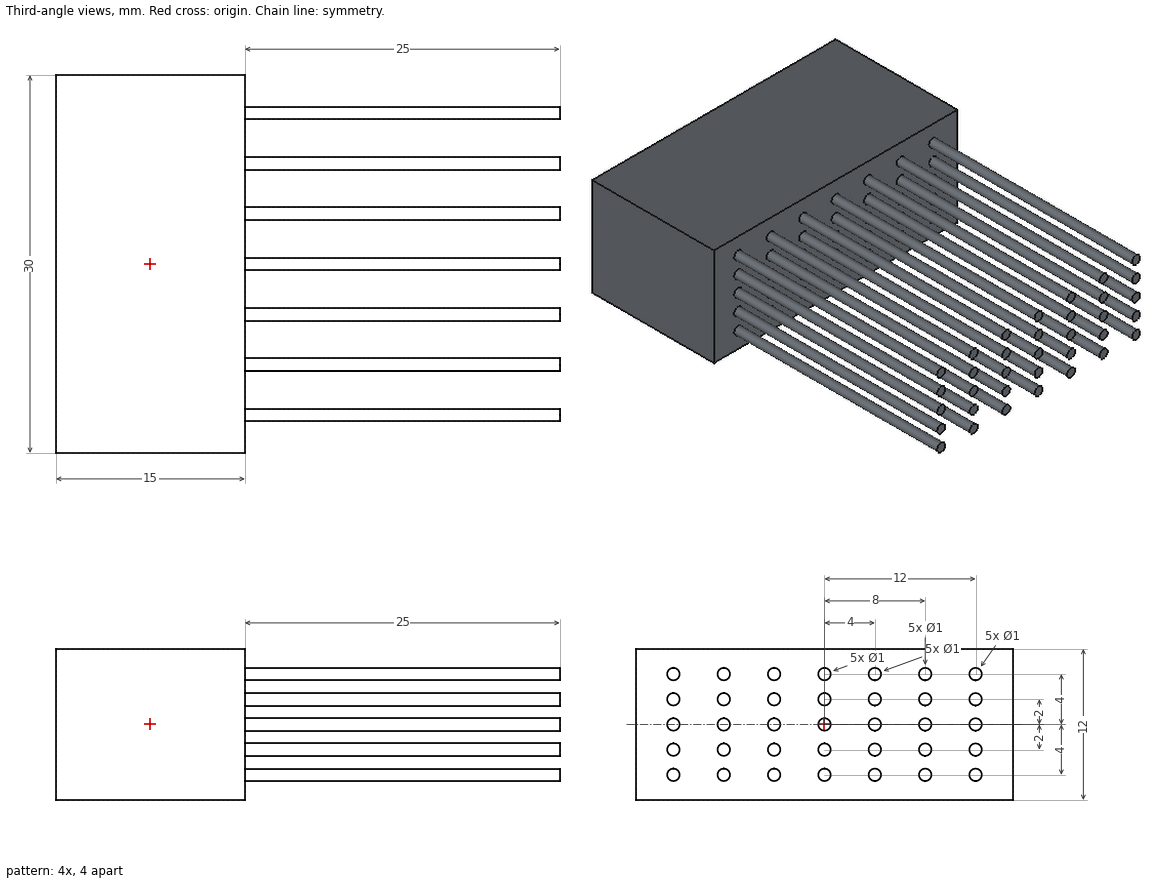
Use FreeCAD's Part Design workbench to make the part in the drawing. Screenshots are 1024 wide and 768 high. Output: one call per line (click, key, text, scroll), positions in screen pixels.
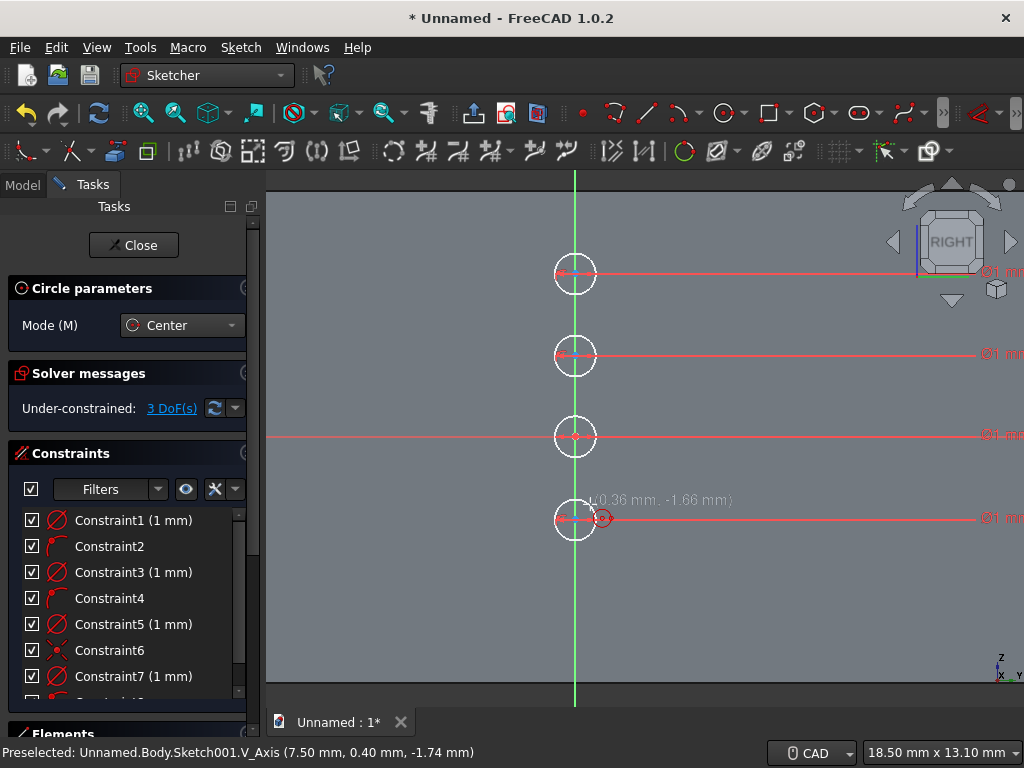
click(575, 601)
move(590, 586)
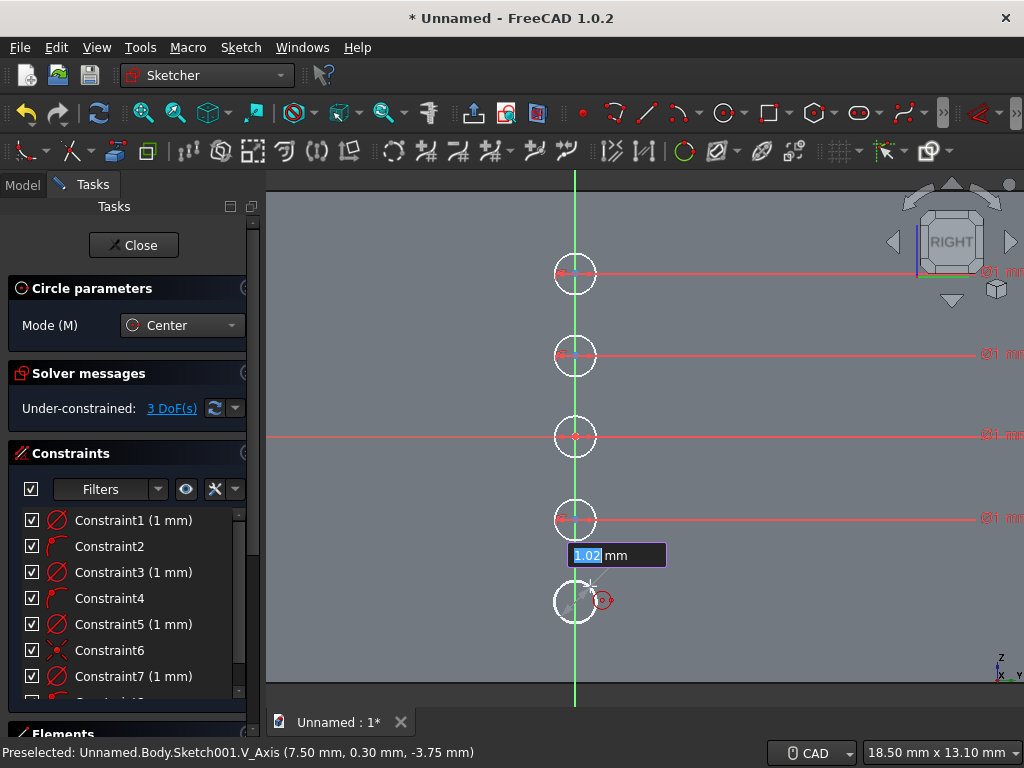
text(1)
key(Return)
key(Escape)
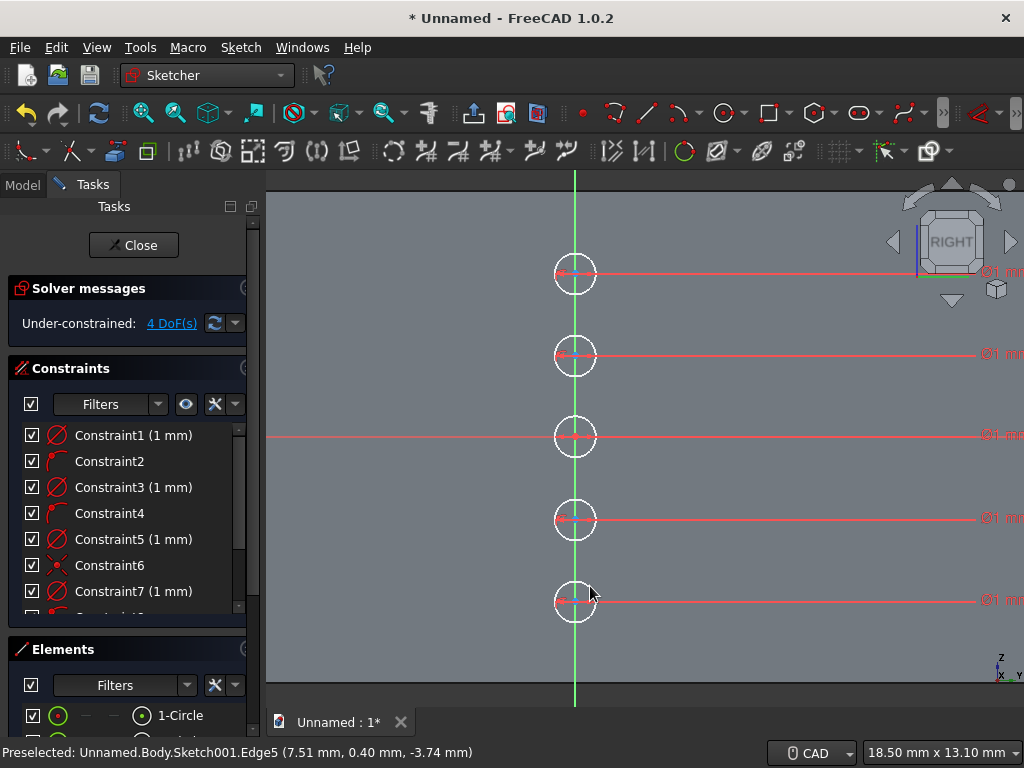
click(575, 274)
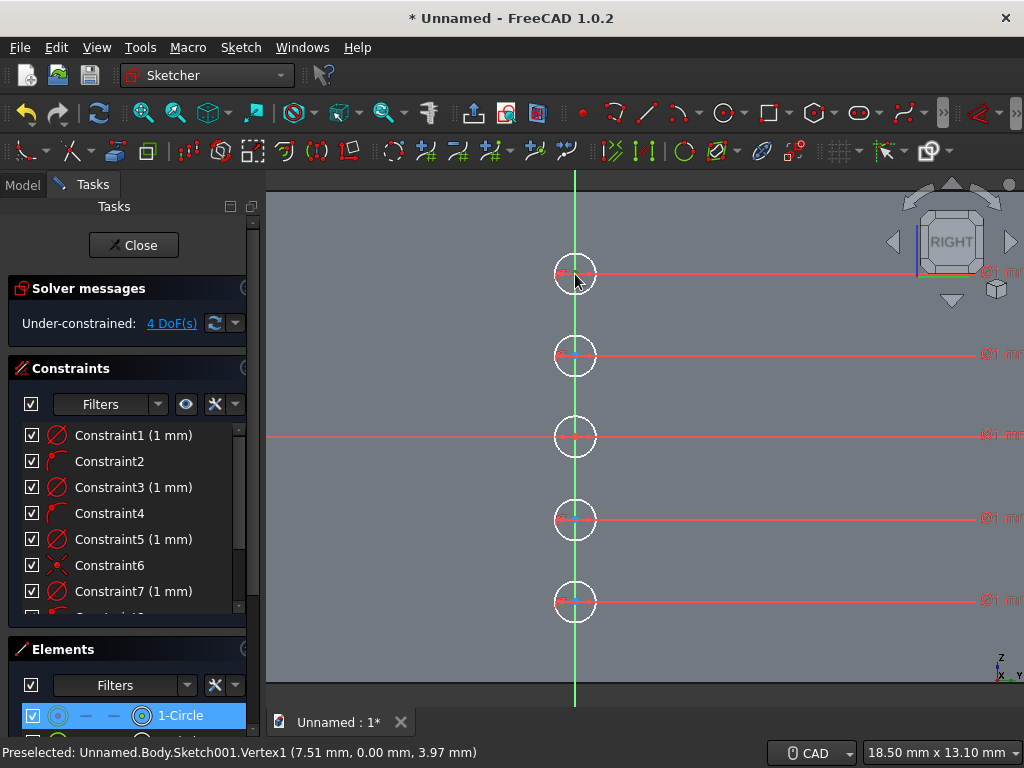
key(i)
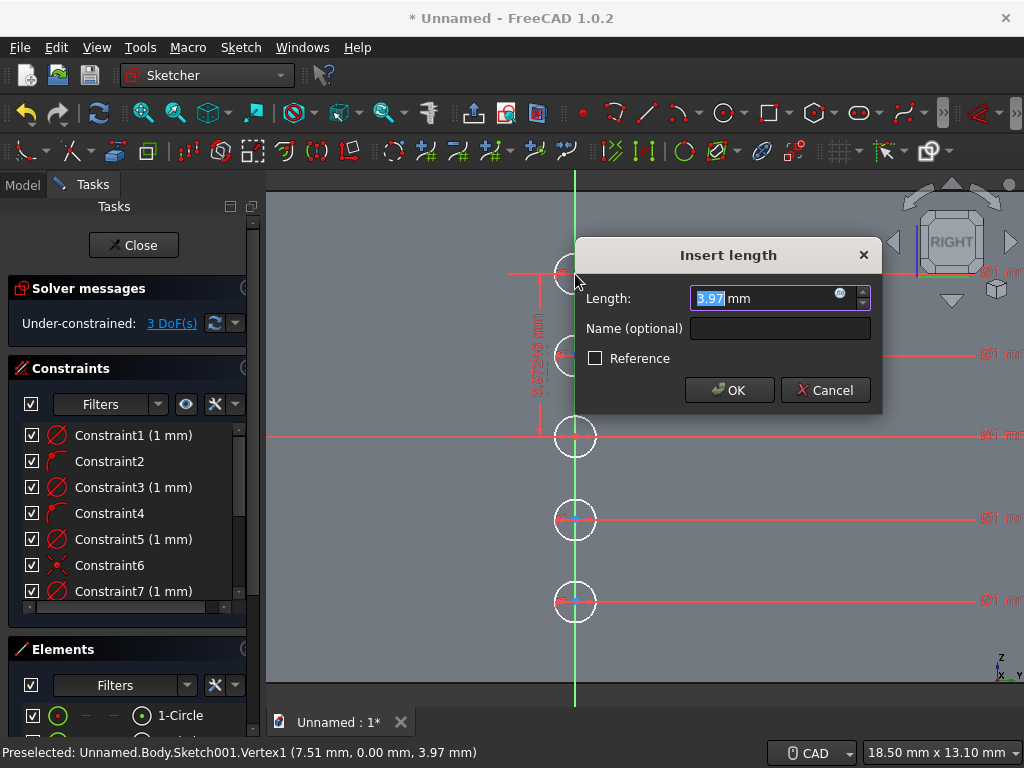
text(4)
key(Return)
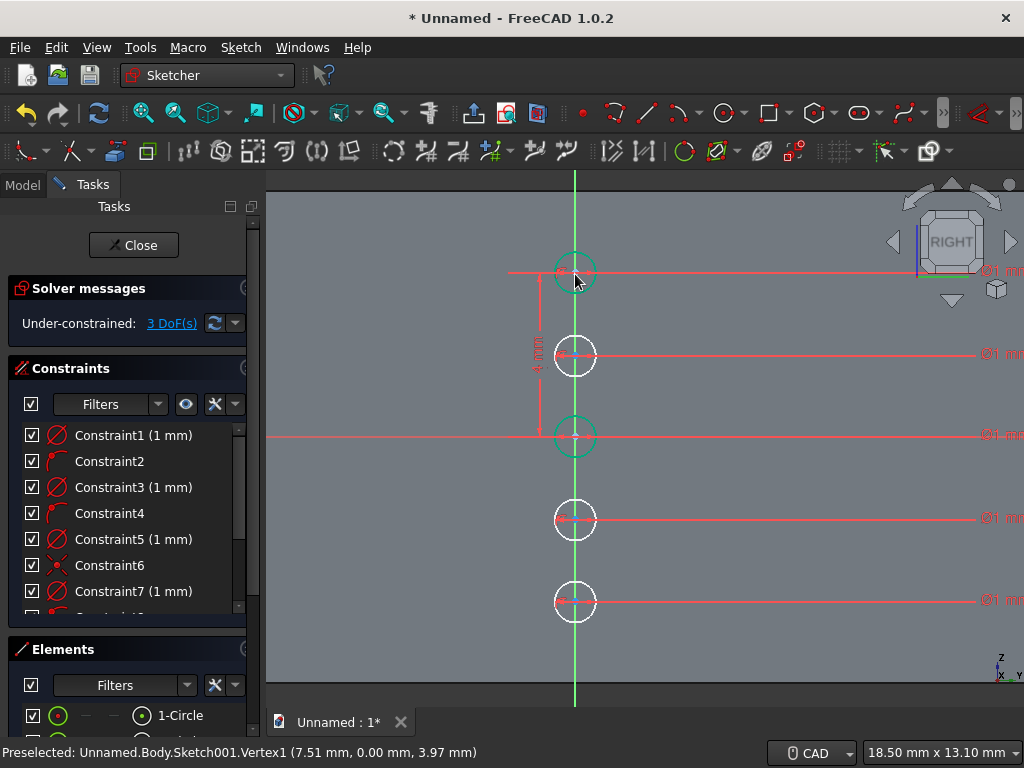
click(575, 356)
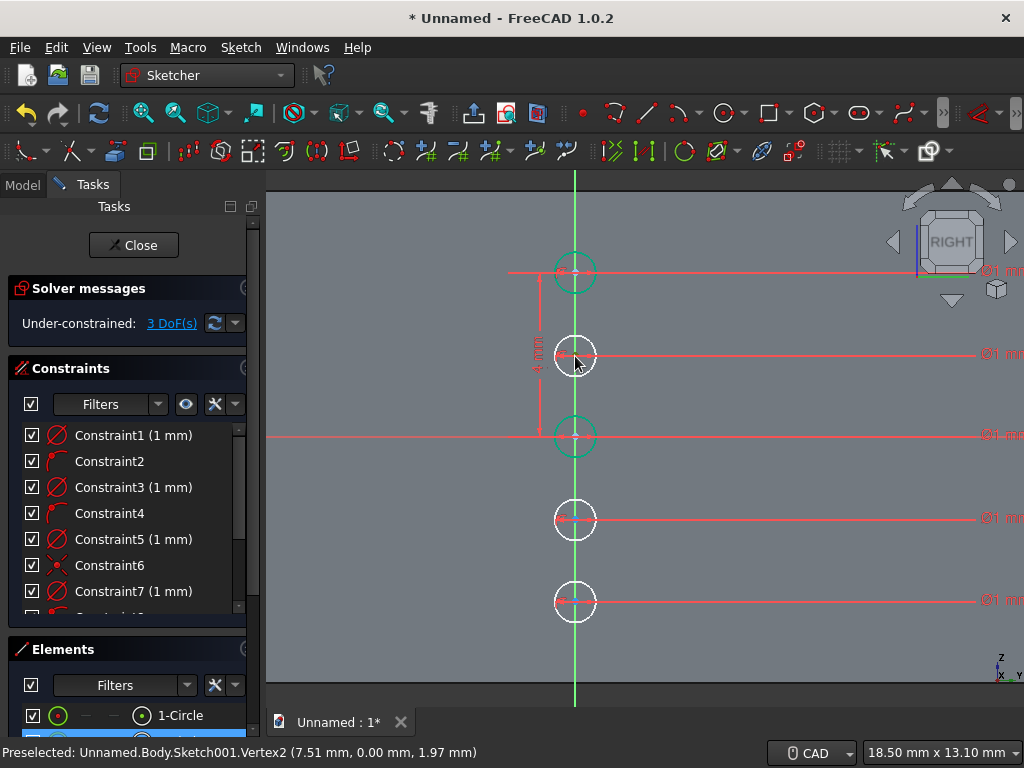
click(1002, 114)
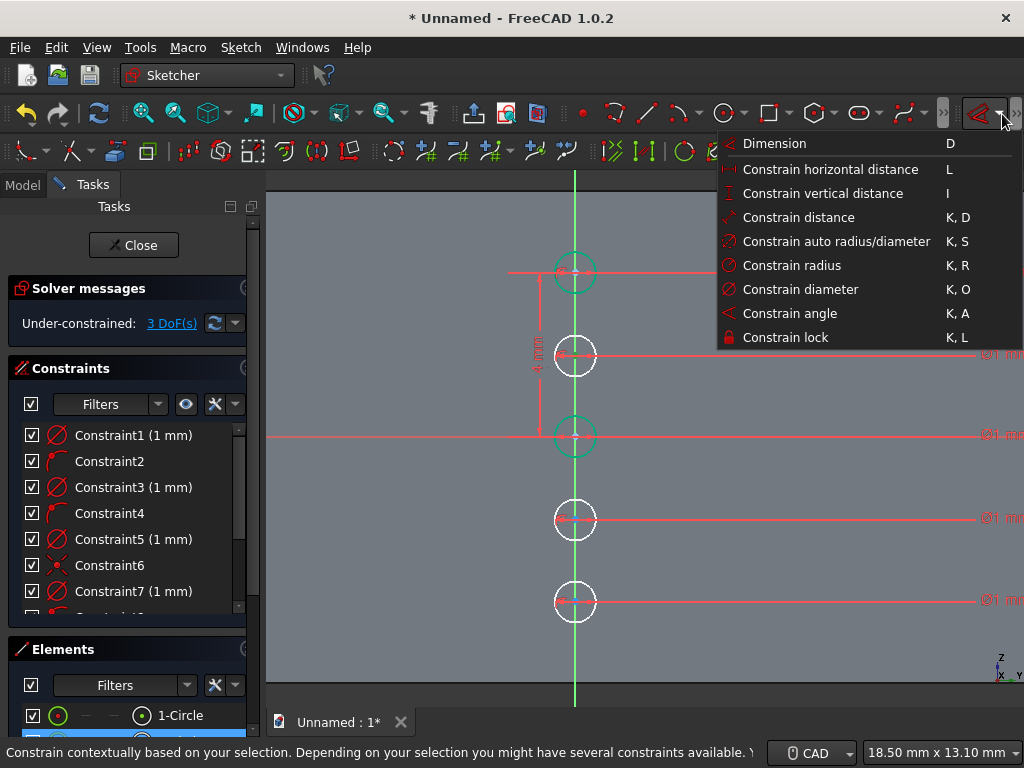
click(870, 193)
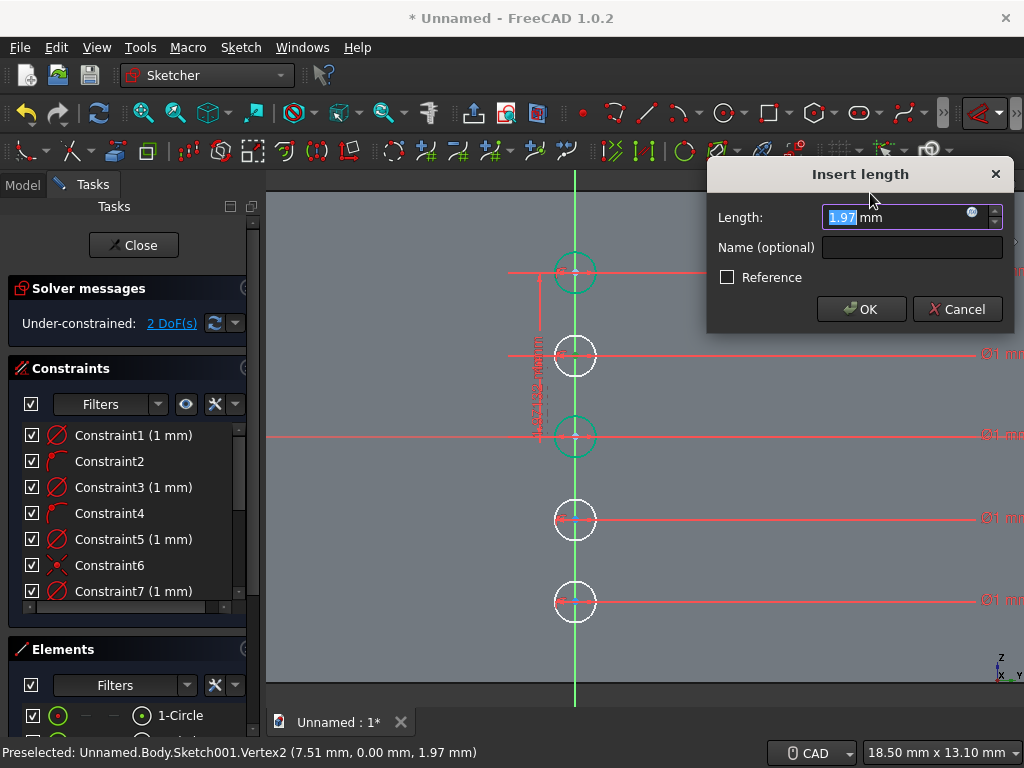
text(2)
key(Return)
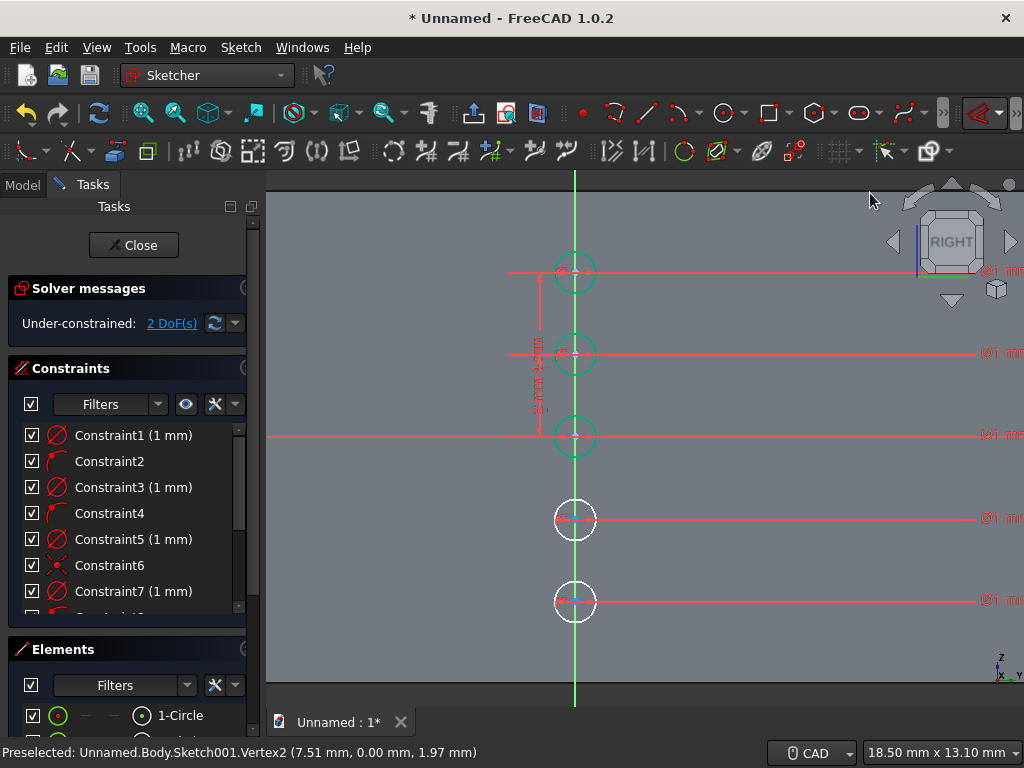
click(575, 520)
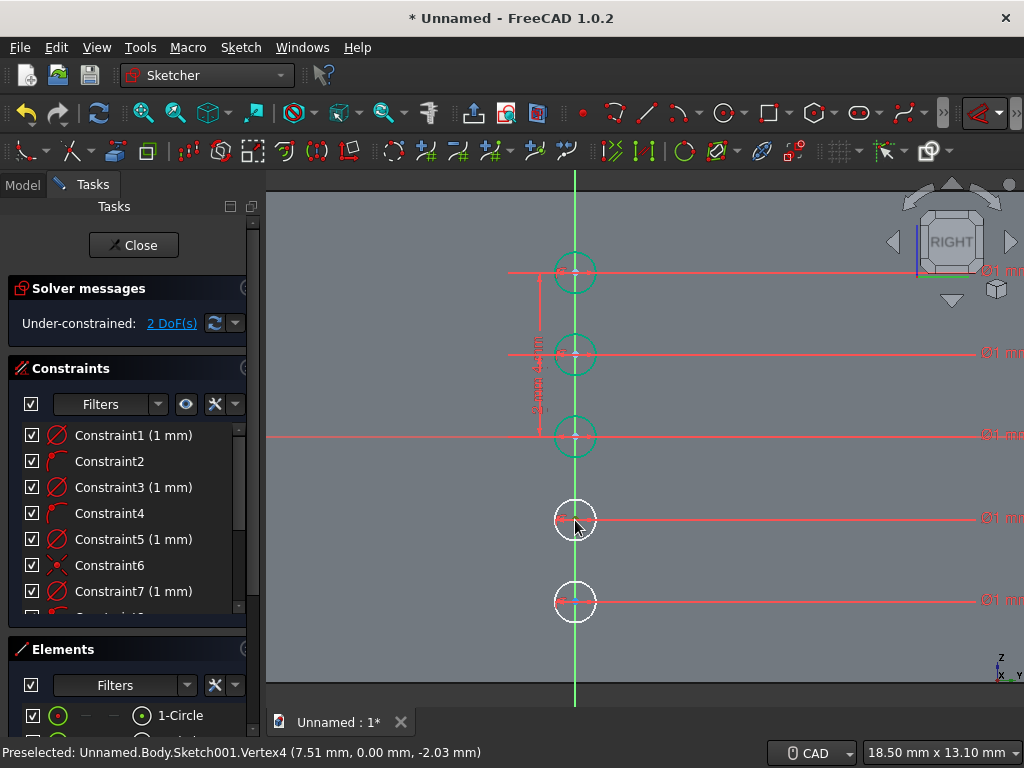
key(i)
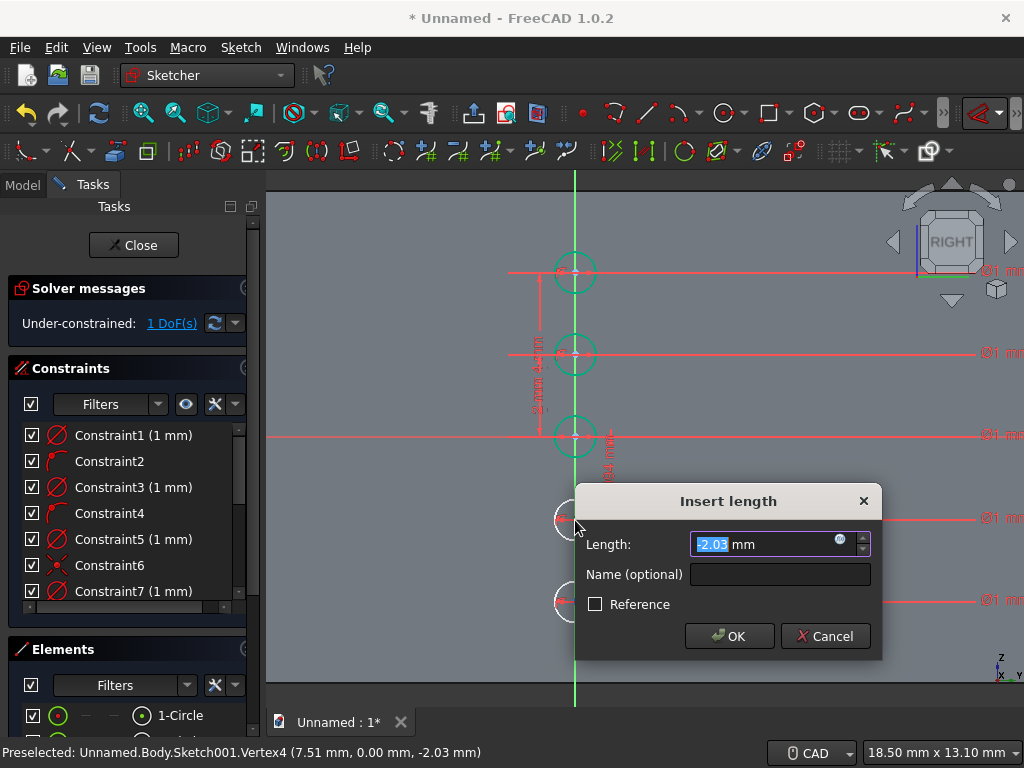
text(-2)
key(Return)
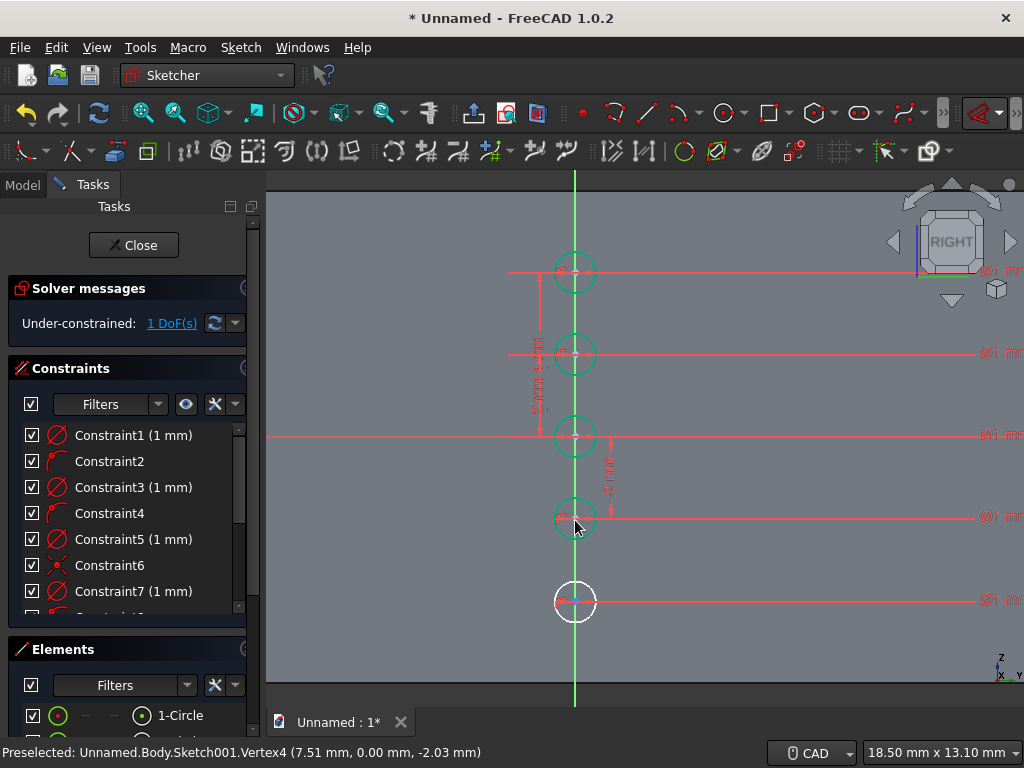
click(575, 602)